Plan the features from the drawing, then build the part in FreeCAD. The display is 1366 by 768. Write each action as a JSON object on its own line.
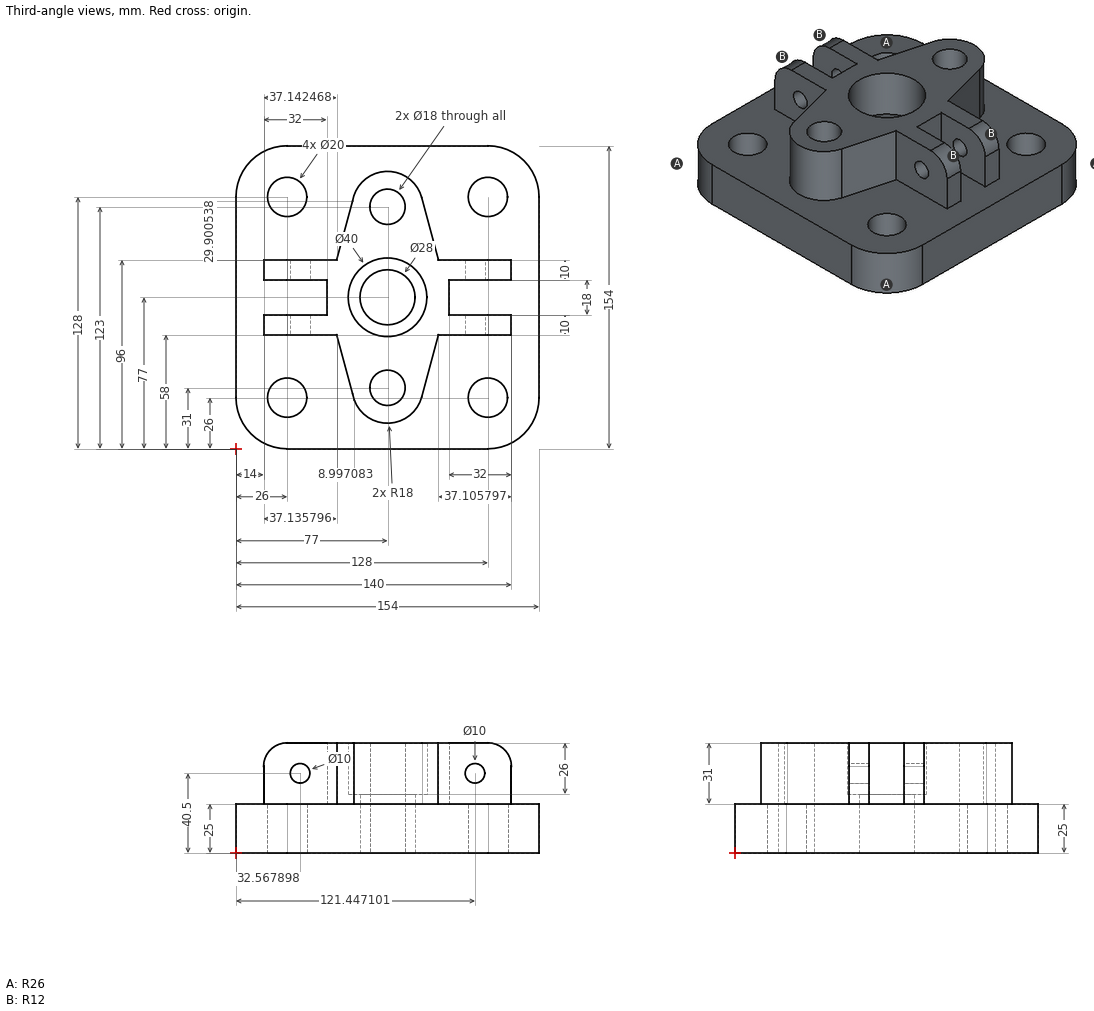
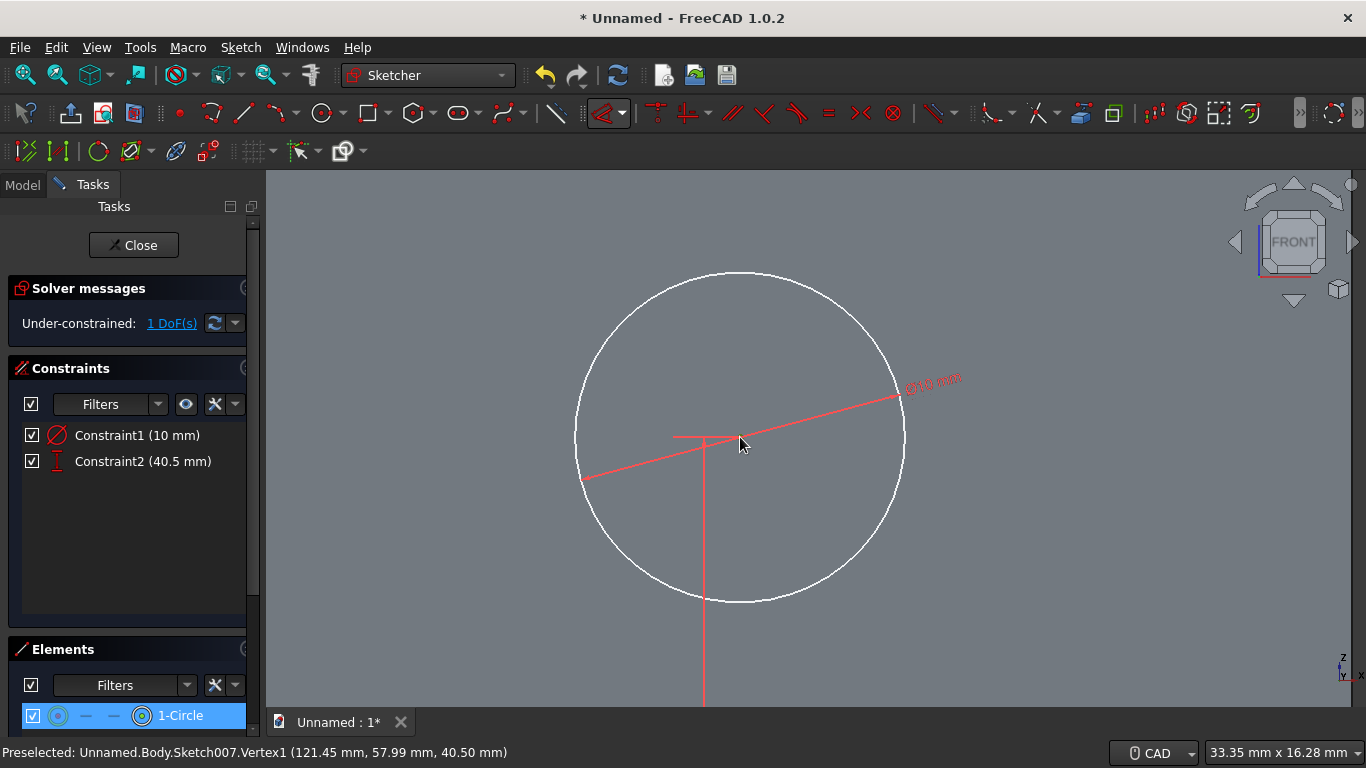
{"action": "left_click", "coordinate": [624, 114]}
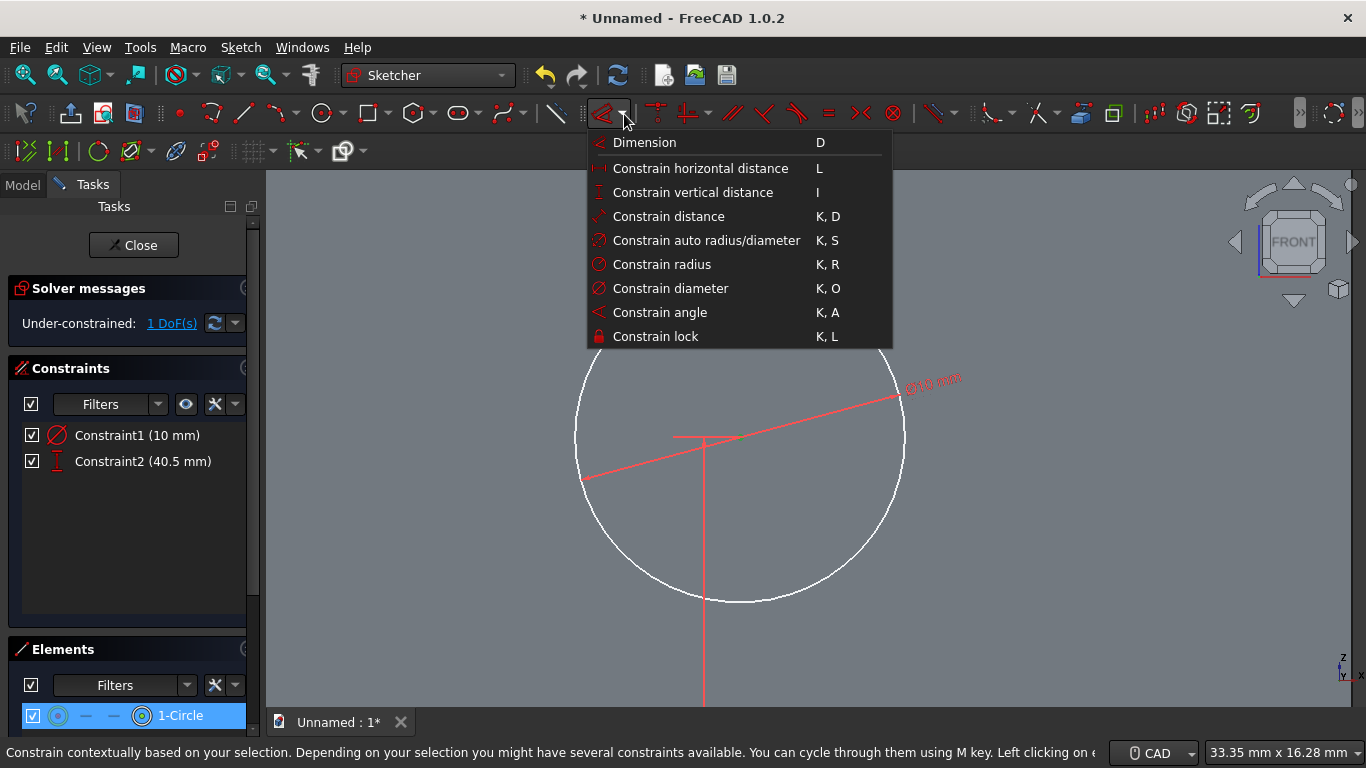
{"action": "left_click", "coordinate": [740, 168]}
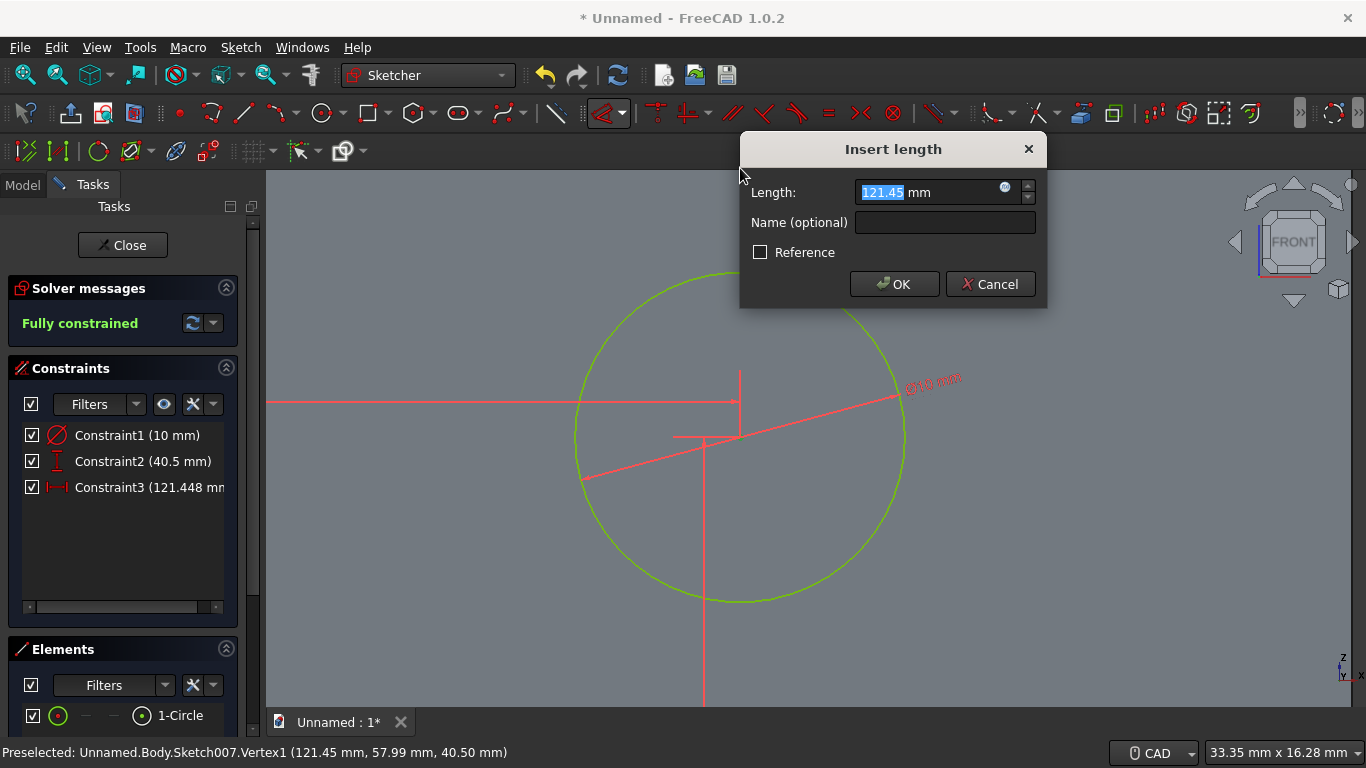
{"action": "type", "text": "121.447101"}
{"action": "key", "text": "Return"}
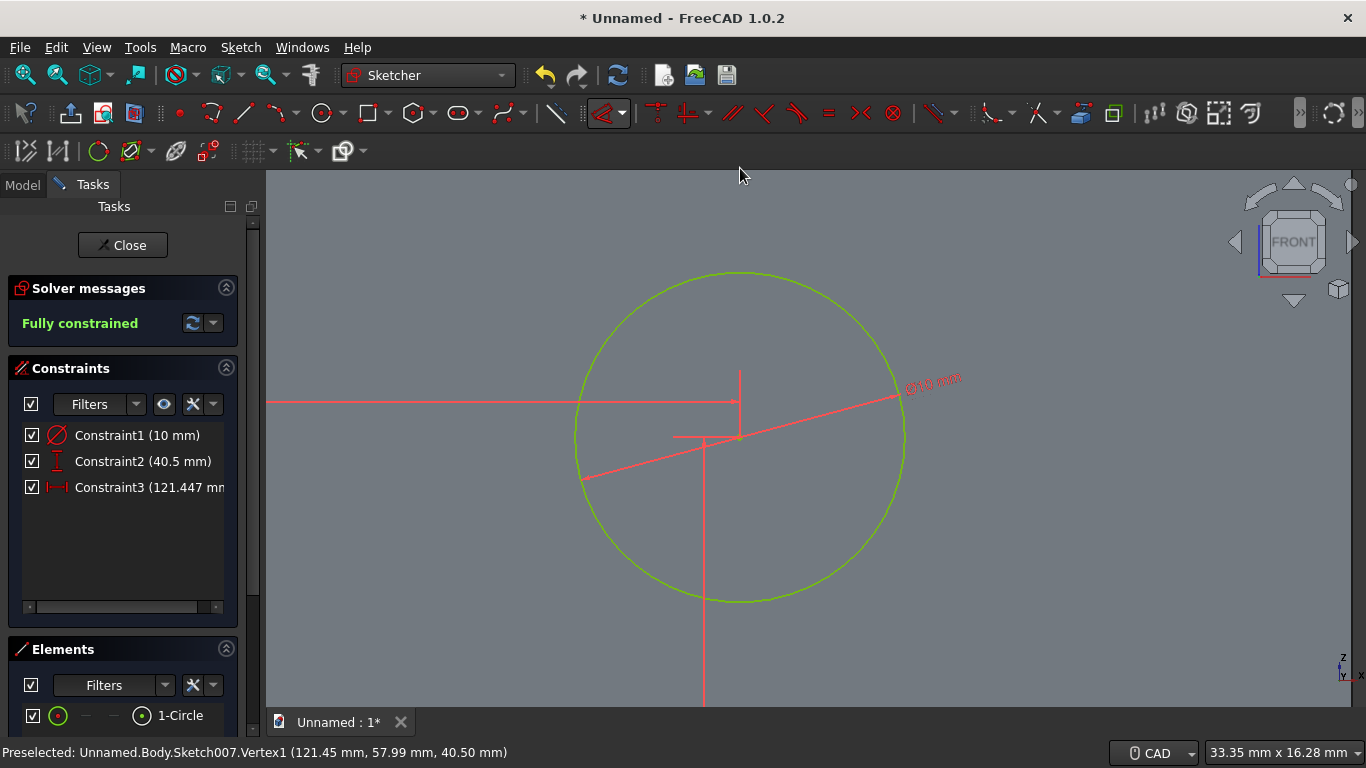
{"action": "left_click", "coordinate": [123, 245]}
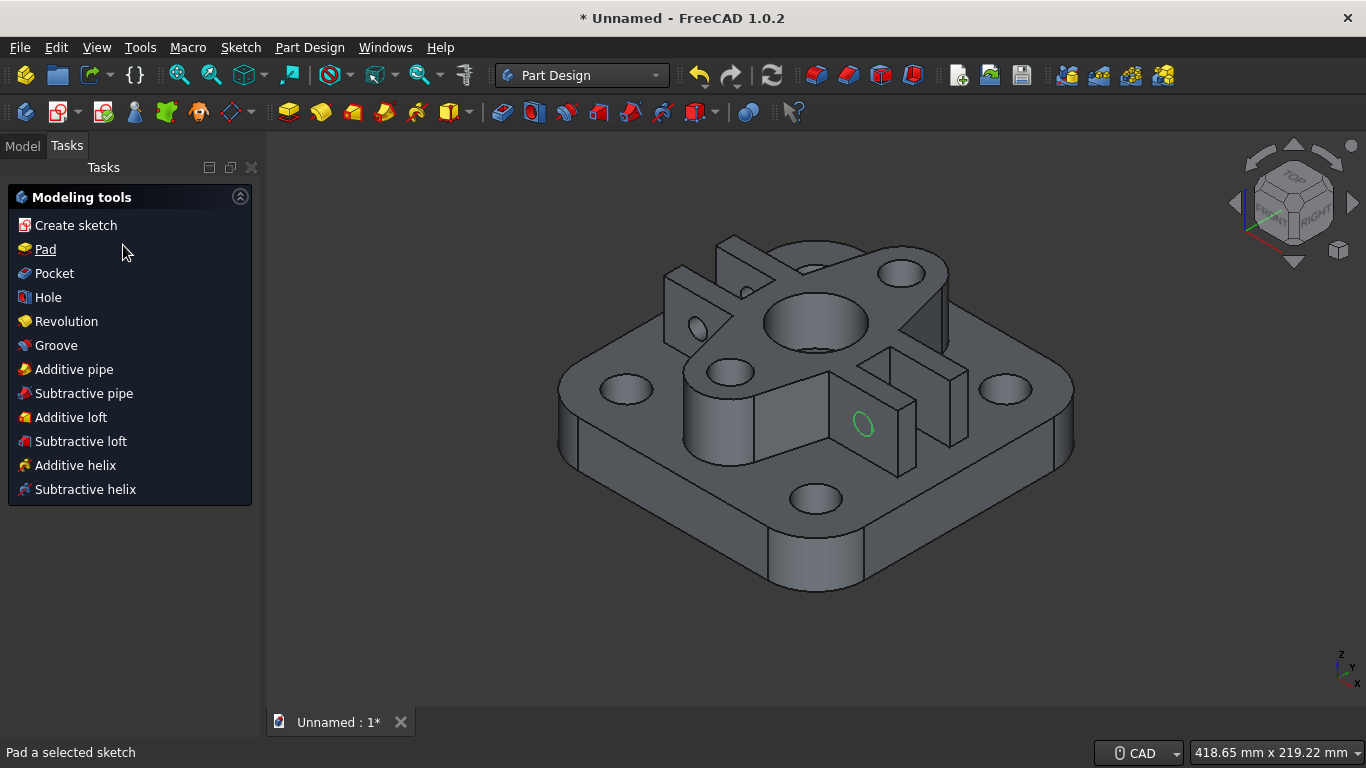
{"action": "left_click", "coordinate": [504, 112]}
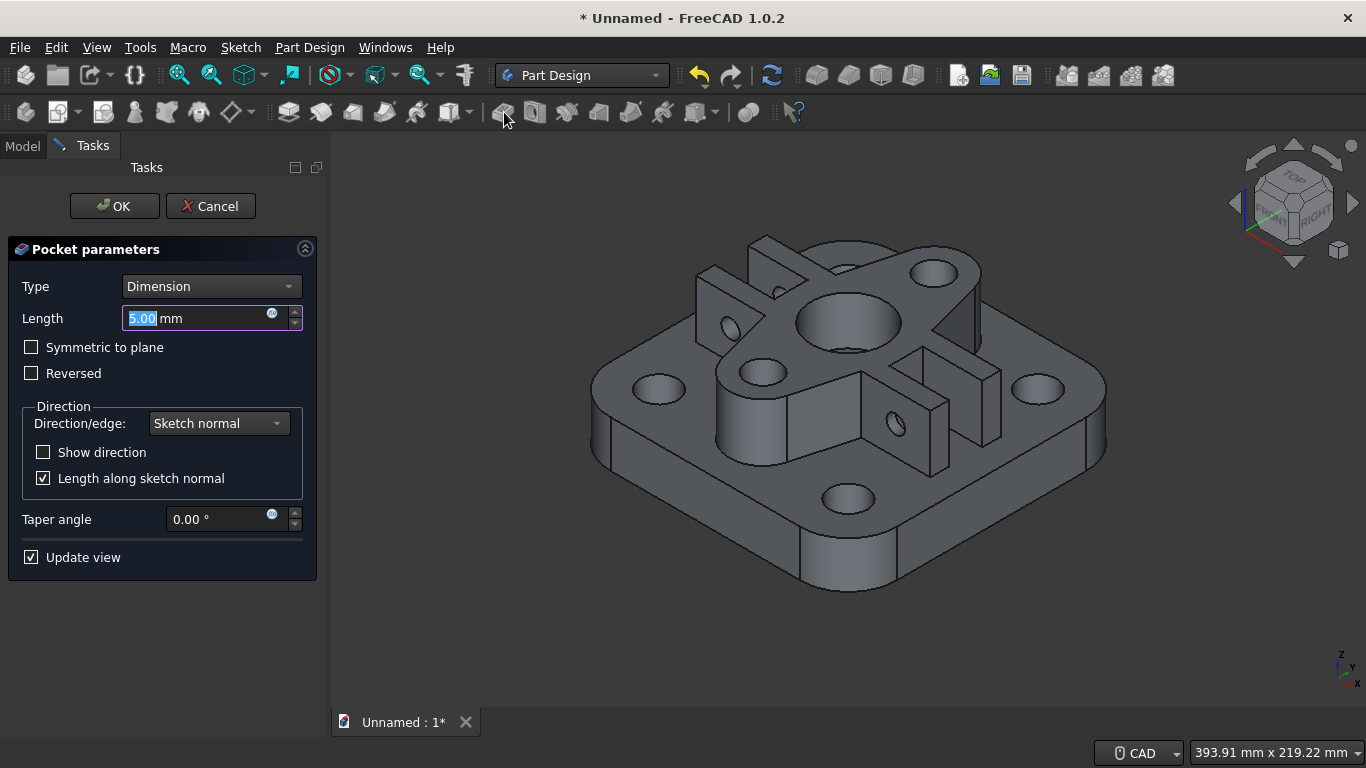
{"action": "left_click", "coordinate": [212, 286]}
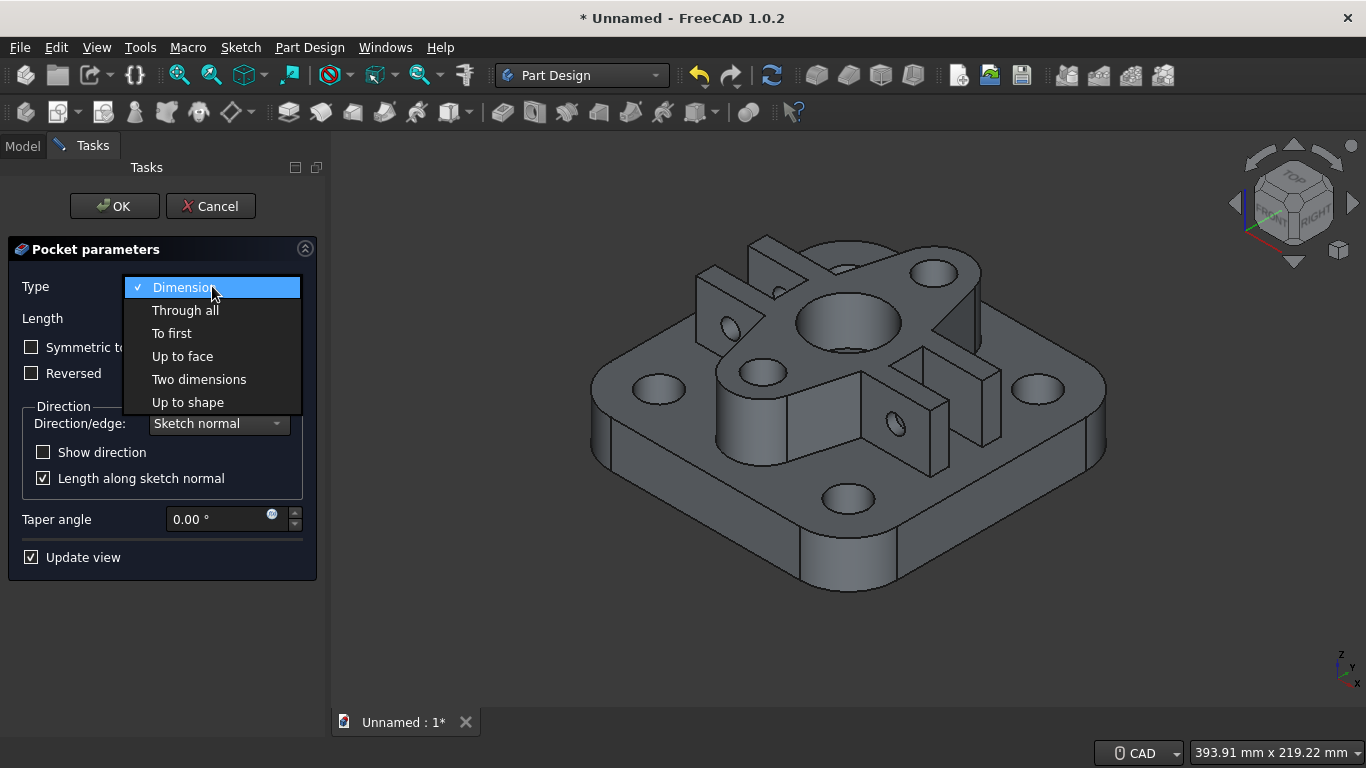
{"action": "left_click", "coordinate": [212, 310]}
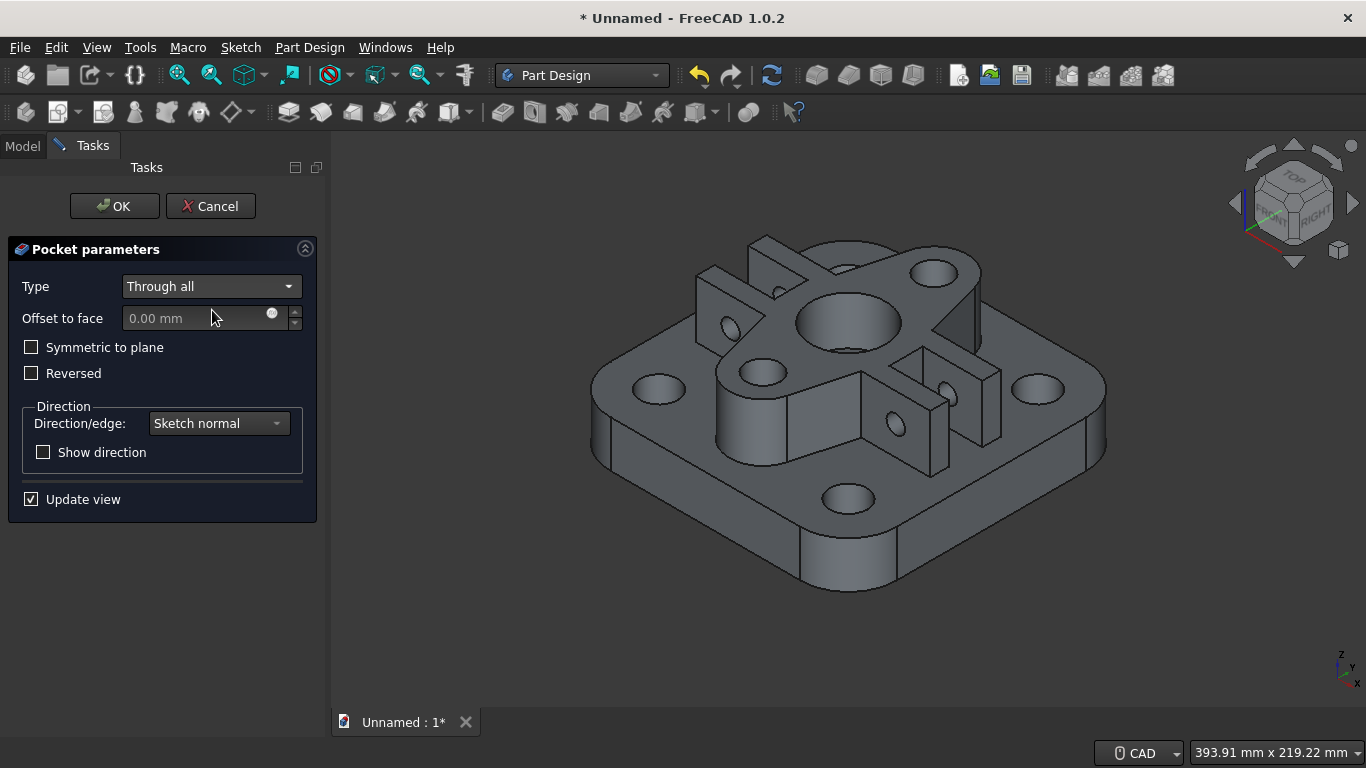
{"action": "left_click", "coordinate": [115, 206]}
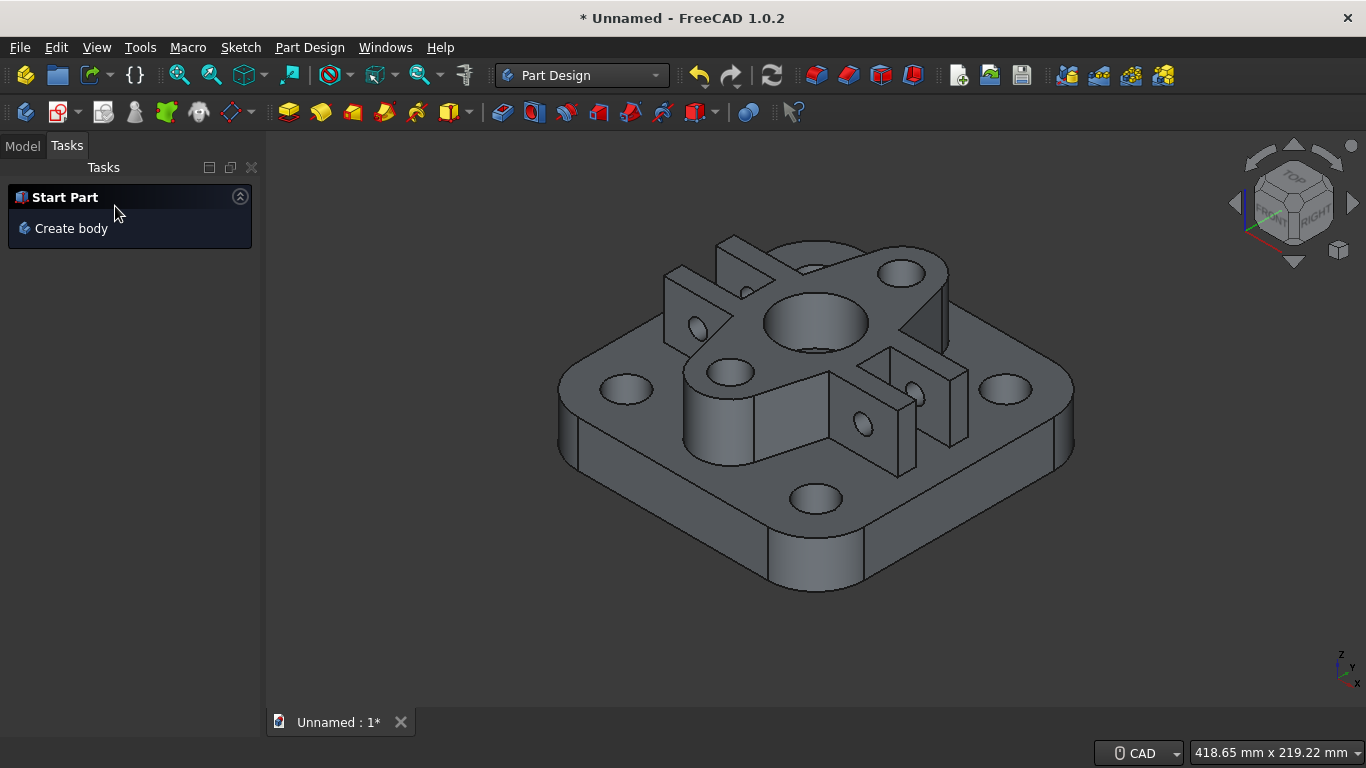
{"action": "left_click", "coordinate": [907, 405]}